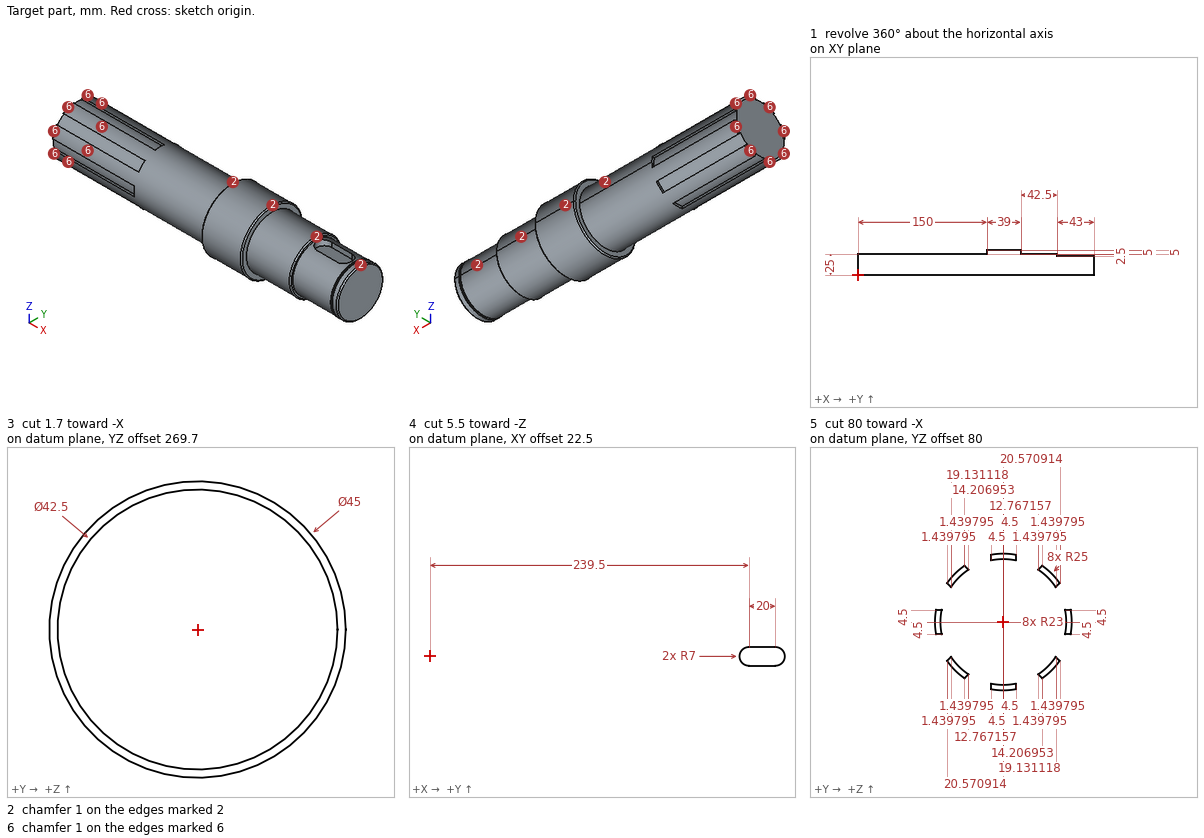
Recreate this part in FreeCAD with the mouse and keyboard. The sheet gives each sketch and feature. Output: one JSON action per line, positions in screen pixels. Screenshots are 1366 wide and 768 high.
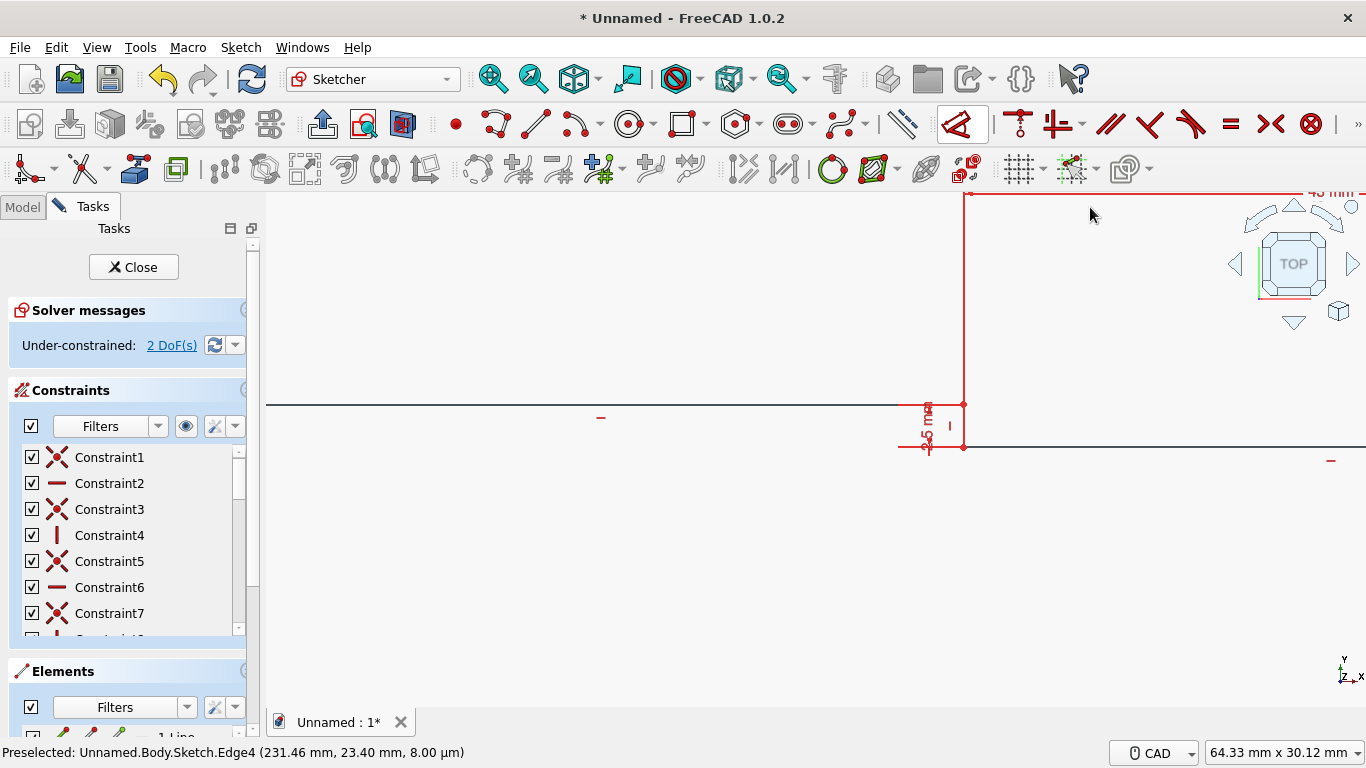
{"action": "scroll", "coordinate": [966, 430], "scroll_direction": "down", "scroll_amount": 10}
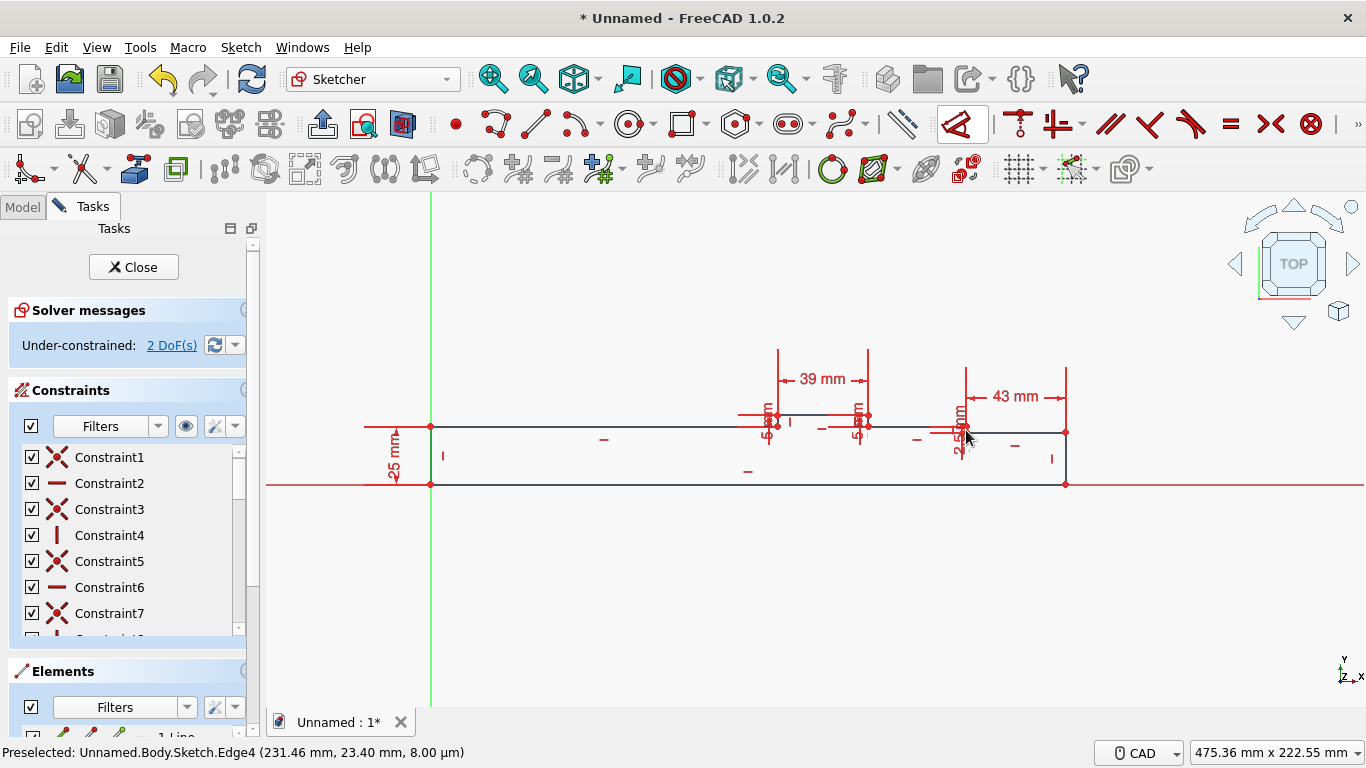
{"action": "left_click", "coordinate": [674, 427]}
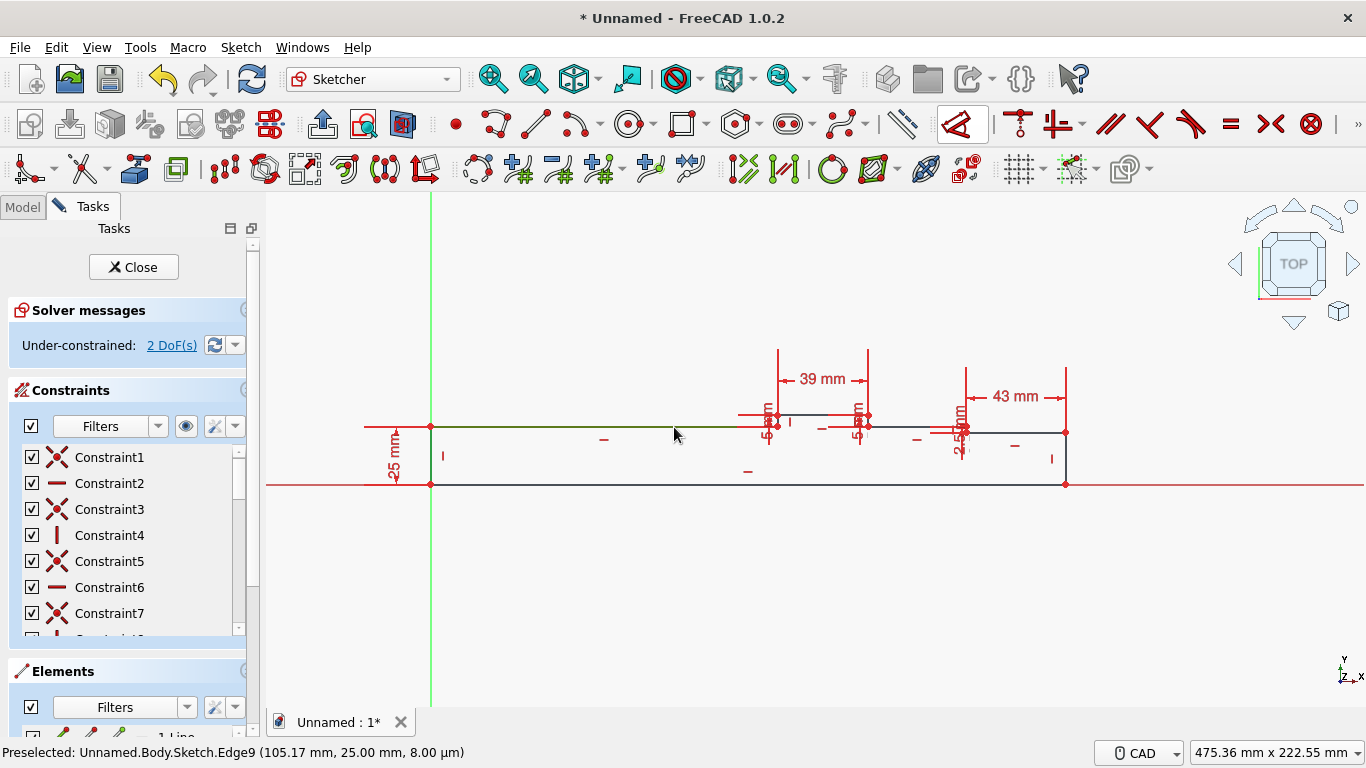
{"action": "key", "text": "l"}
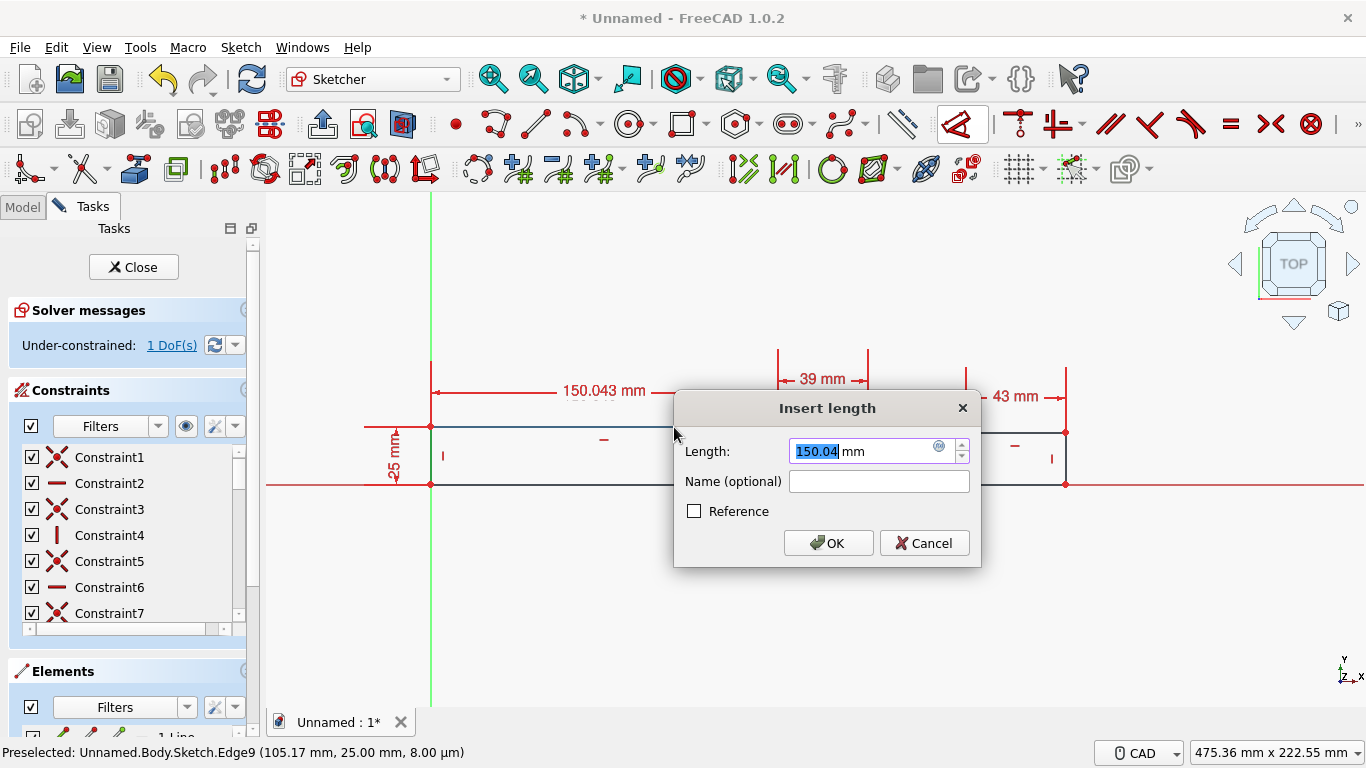
{"action": "type", "text": "150"}
{"action": "key", "text": "Return"}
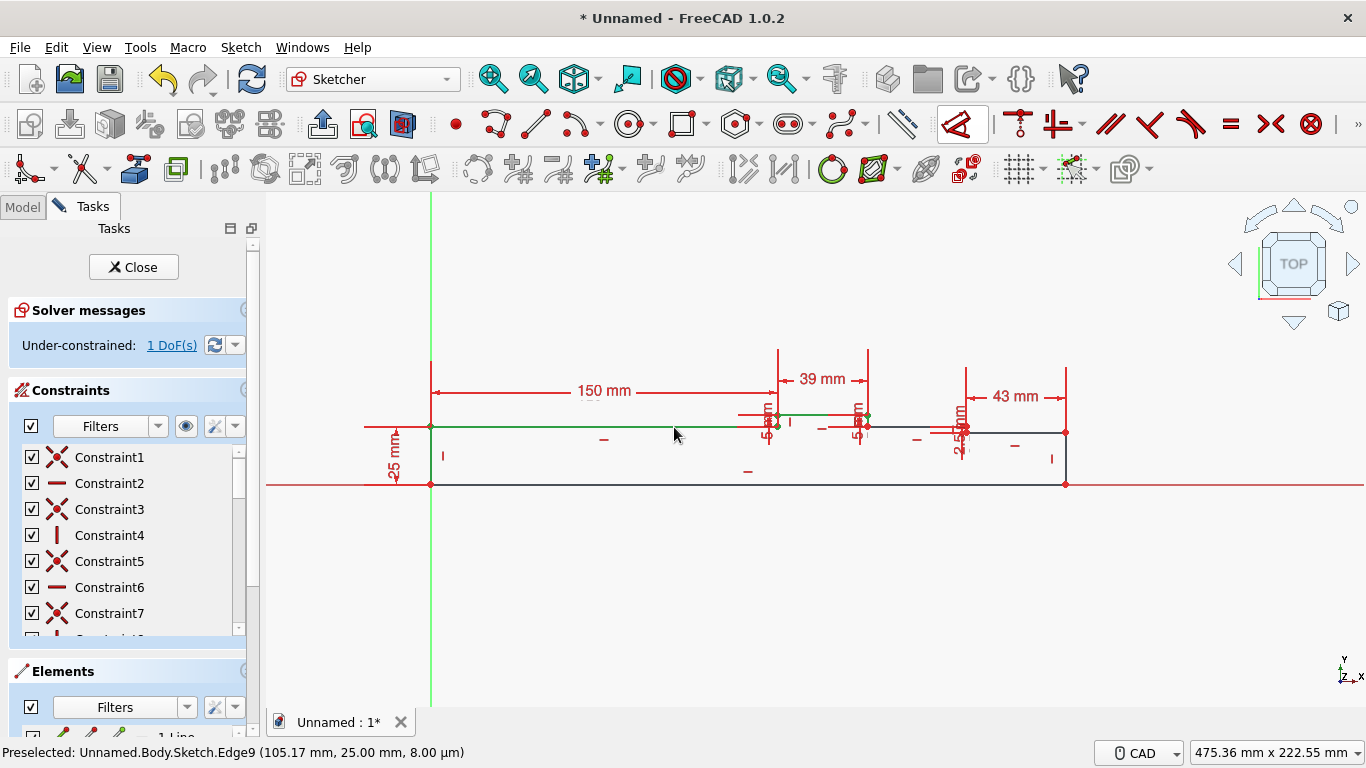
{"action": "left_click", "coordinate": [937, 427]}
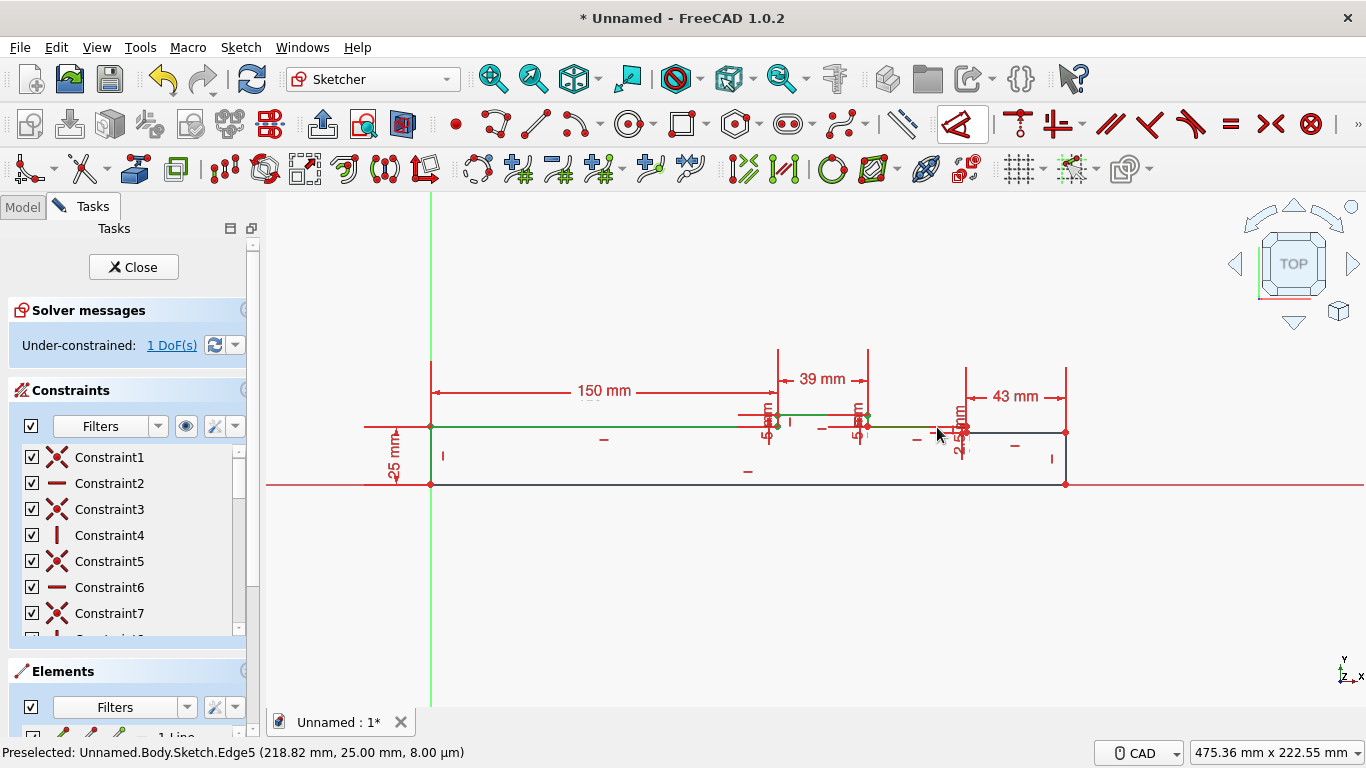
{"action": "key", "text": "l"}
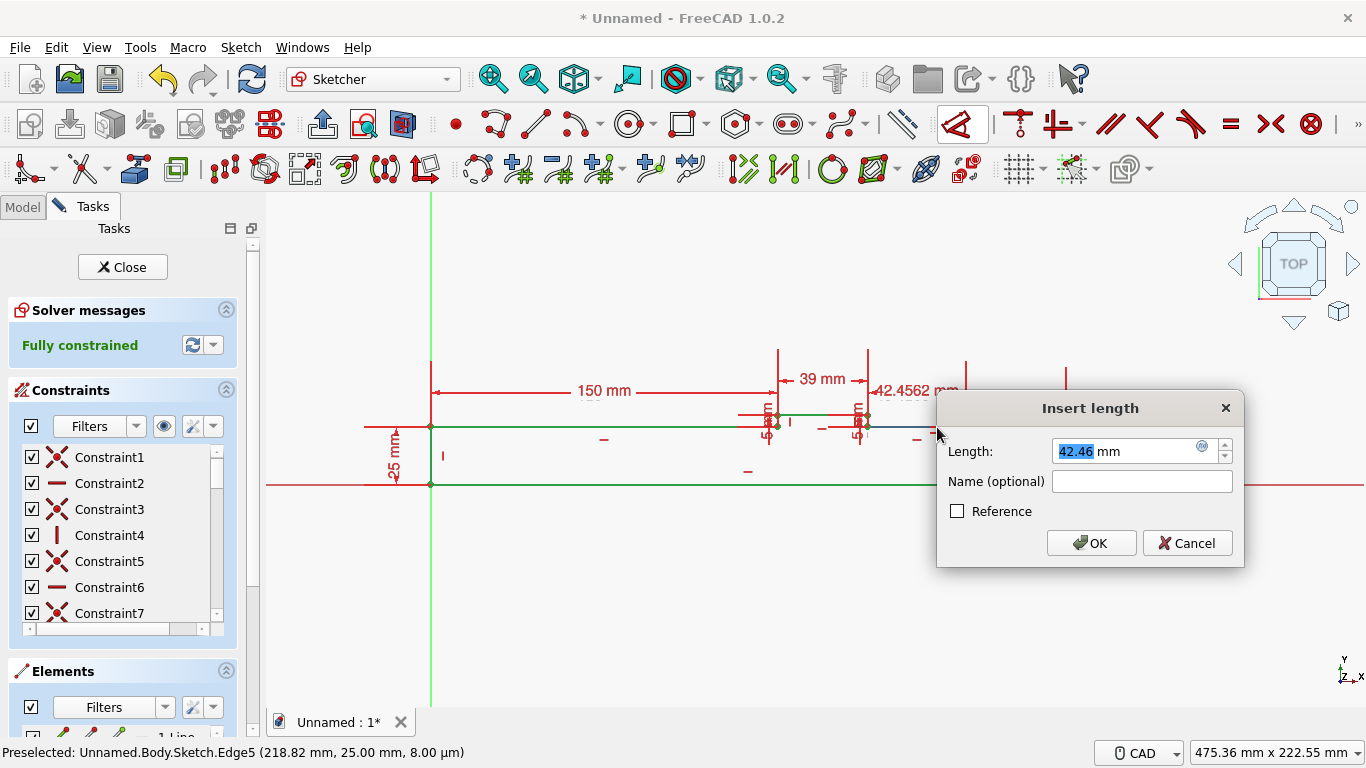
{"action": "type", "text": "42.5"}
{"action": "key", "text": "Return"}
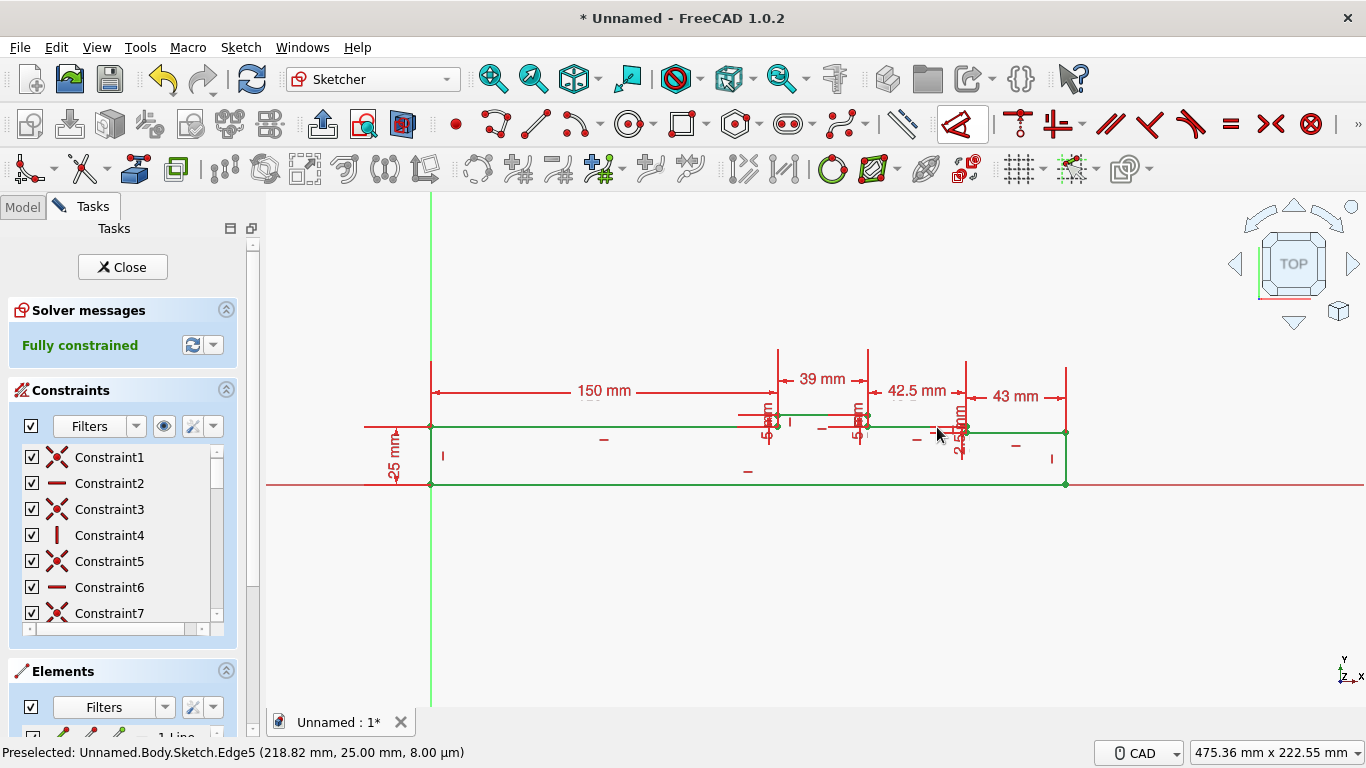
{"action": "left_click", "coordinate": [123, 267]}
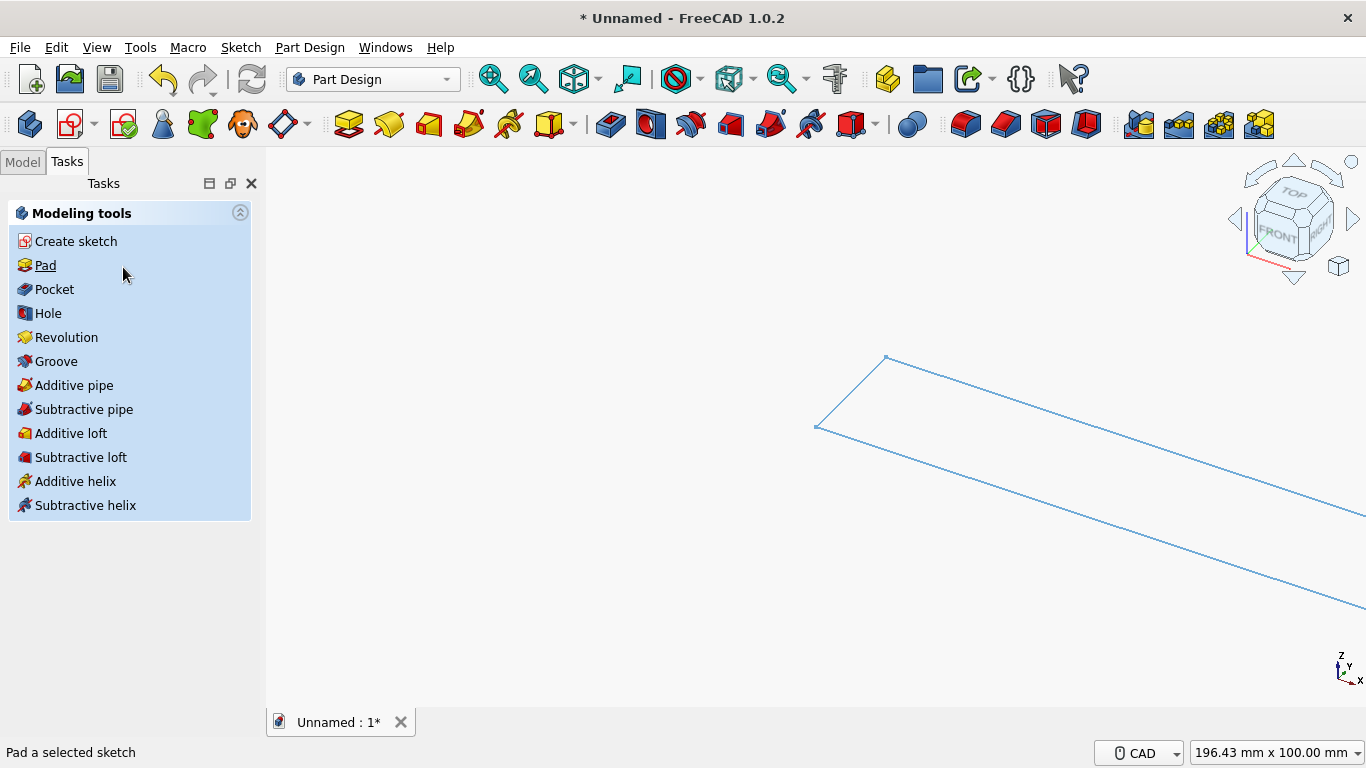
{"action": "left_click", "coordinate": [390, 124]}